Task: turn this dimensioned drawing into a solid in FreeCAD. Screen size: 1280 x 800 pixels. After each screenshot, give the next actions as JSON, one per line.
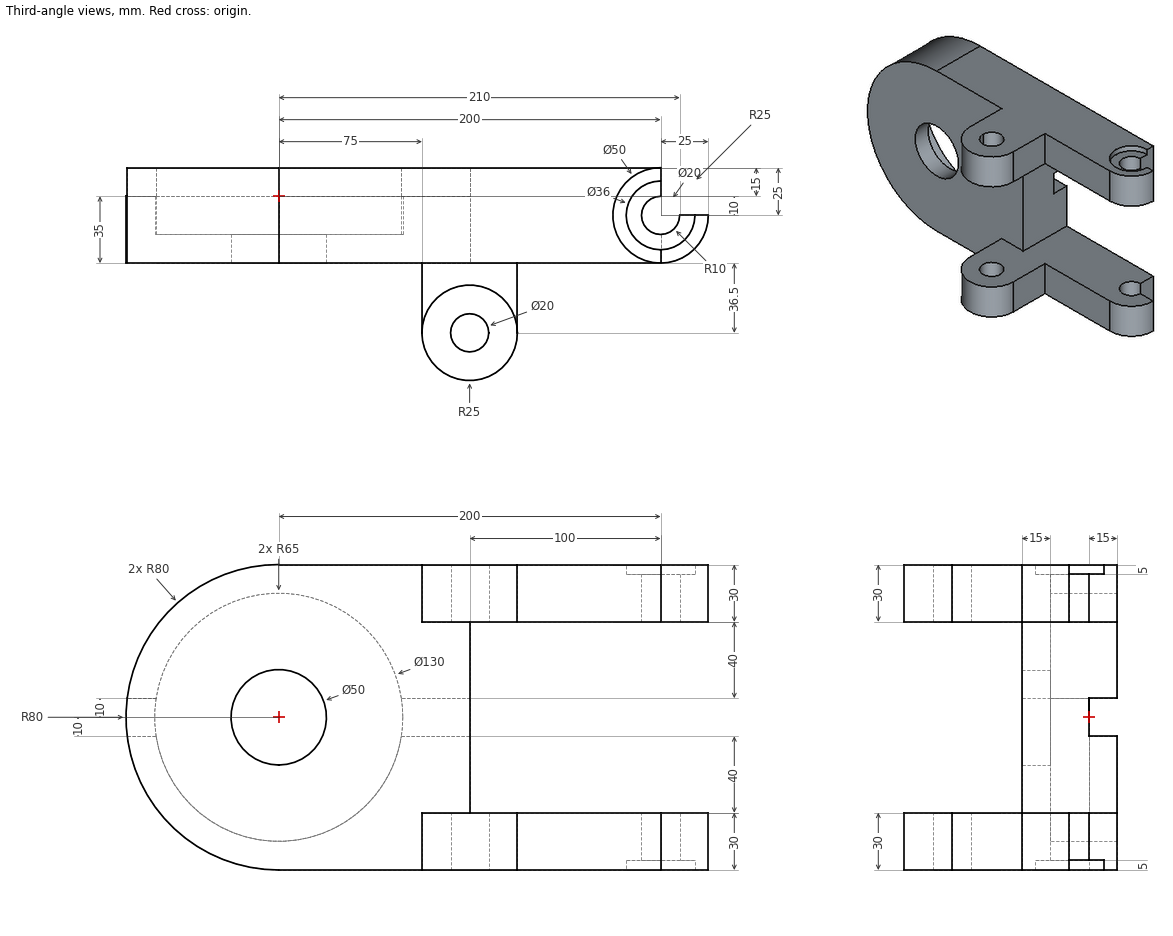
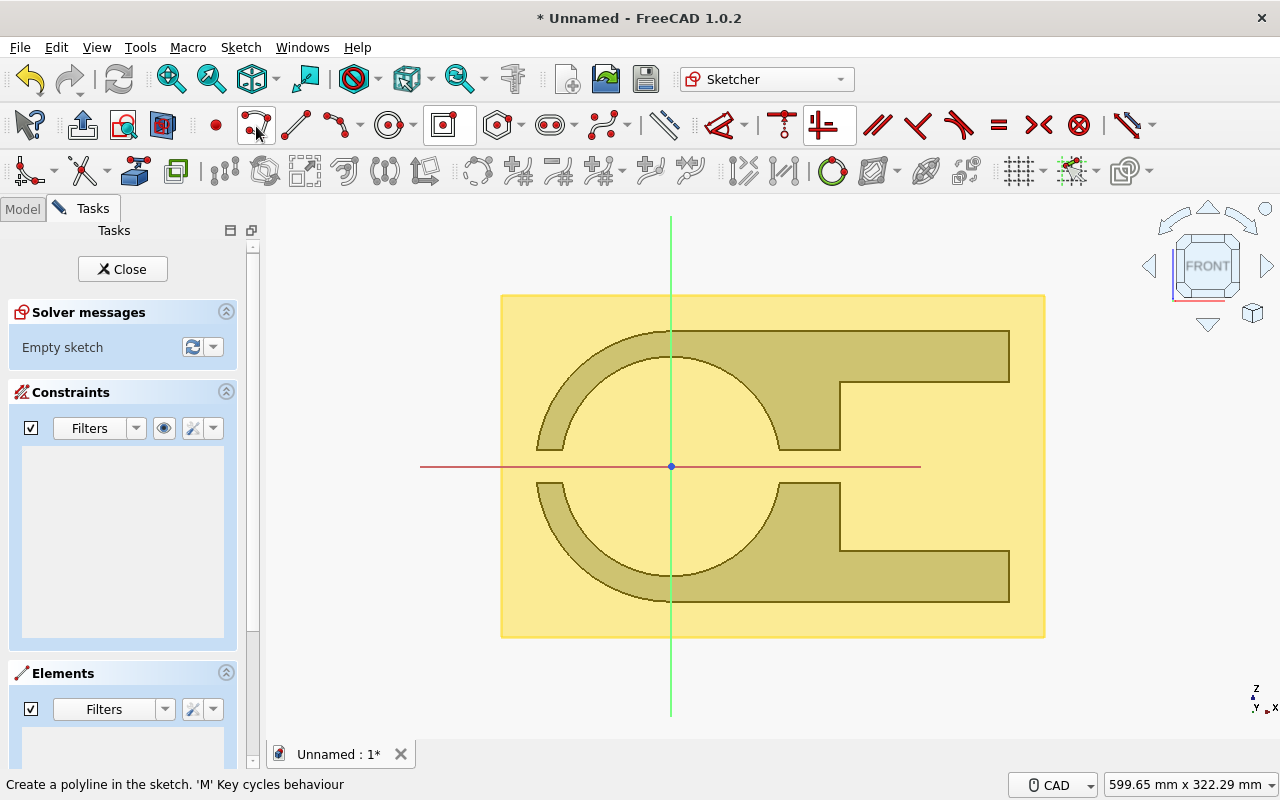
{"action": "left_click", "coordinate": [671, 602]}
{"action": "left_click", "coordinate": [1009, 602]}
{"action": "left_click", "coordinate": [1009, 551]}
{"action": "left_click", "coordinate": [840, 551]}
{"action": "left_click", "coordinate": [840, 382]}
{"action": "left_click", "coordinate": [1009, 382]}
{"action": "left_click", "coordinate": [1009, 331]}
{"action": "left_click", "coordinate": [671, 331]}
{"action": "right_click", "coordinate": [671, 331]}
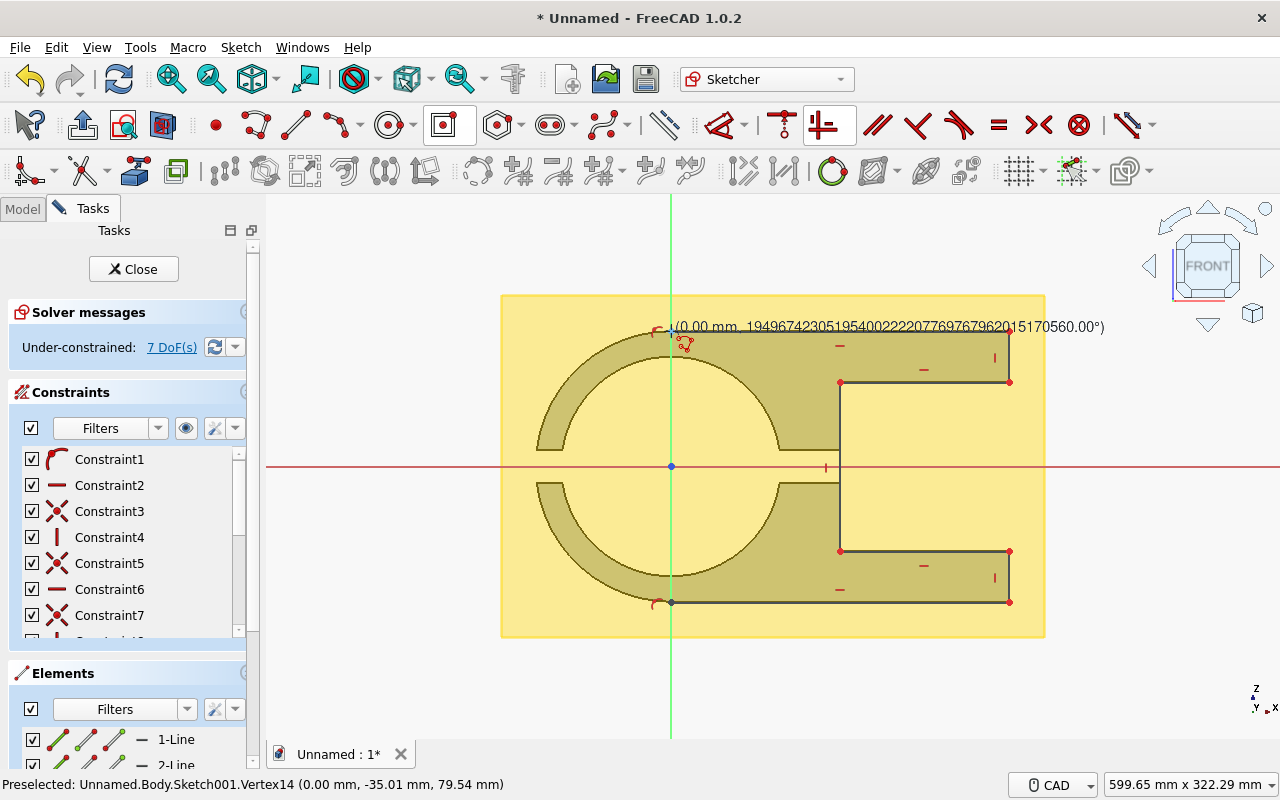
{"action": "left_click", "coordinate": [336, 126]}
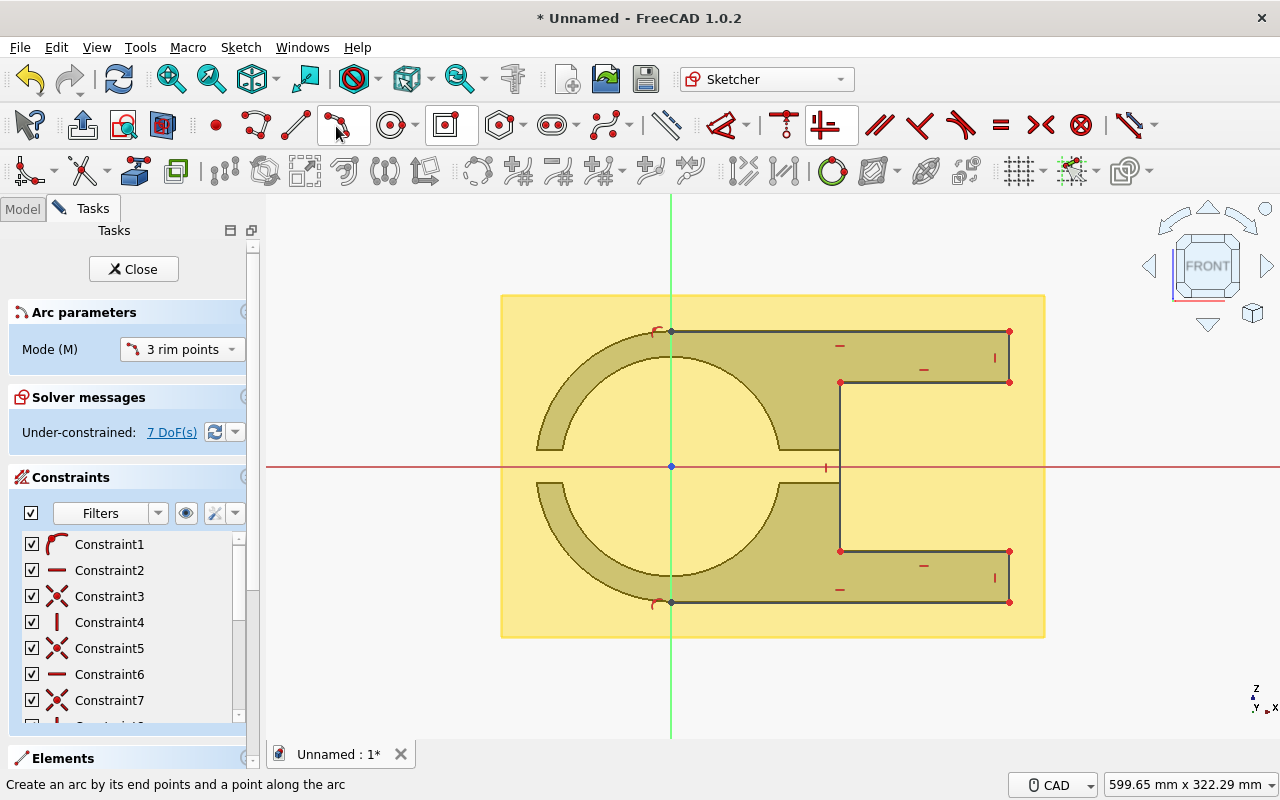
{"action": "left_click", "coordinate": [671, 332]}
{"action": "left_click", "coordinate": [671, 603]}
{"action": "left_click", "coordinate": [542, 425]}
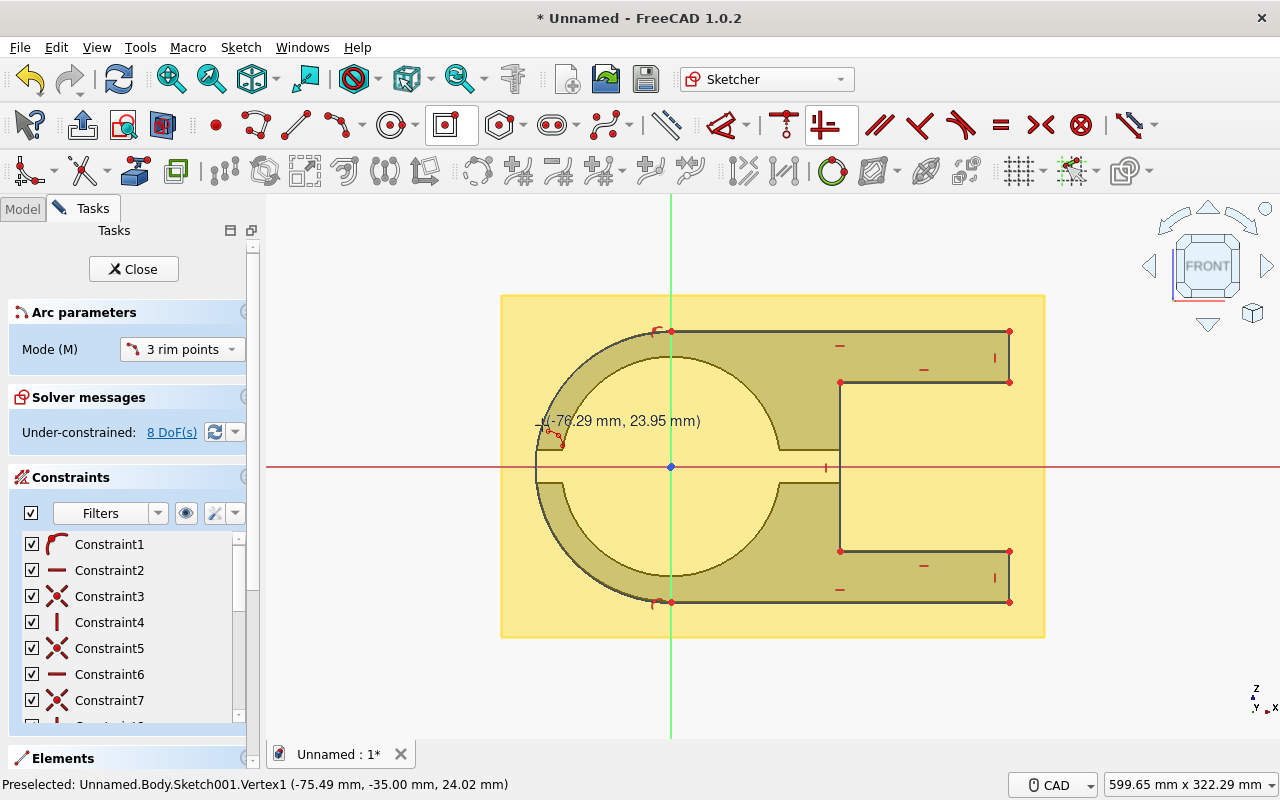
{"action": "left_click", "coordinate": [392, 126]}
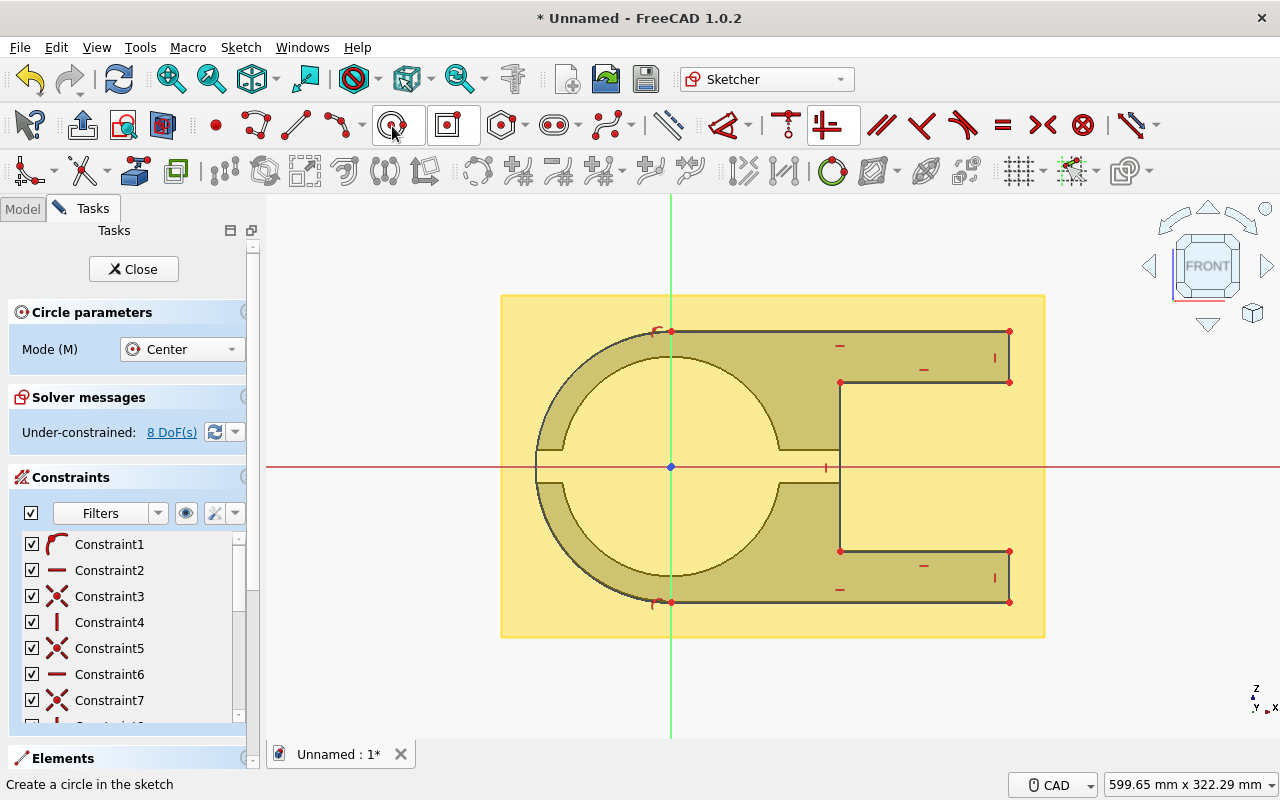
{"action": "left_click", "coordinate": [671, 466]}
{"action": "left_click", "coordinate": [749, 389]}
{"action": "key", "text": "Escape"}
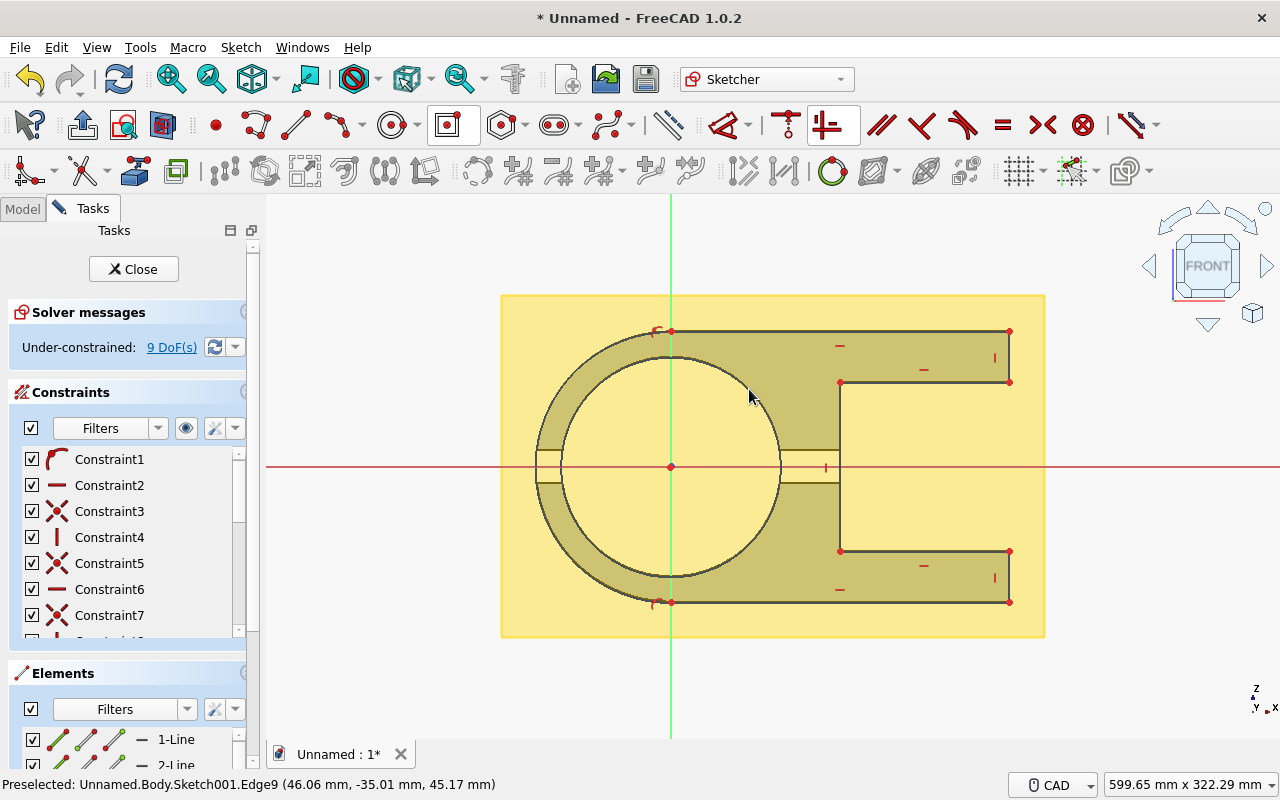
{"action": "left_click_drag", "start_coordinate": [661, 456], "coordinate": [681, 478]}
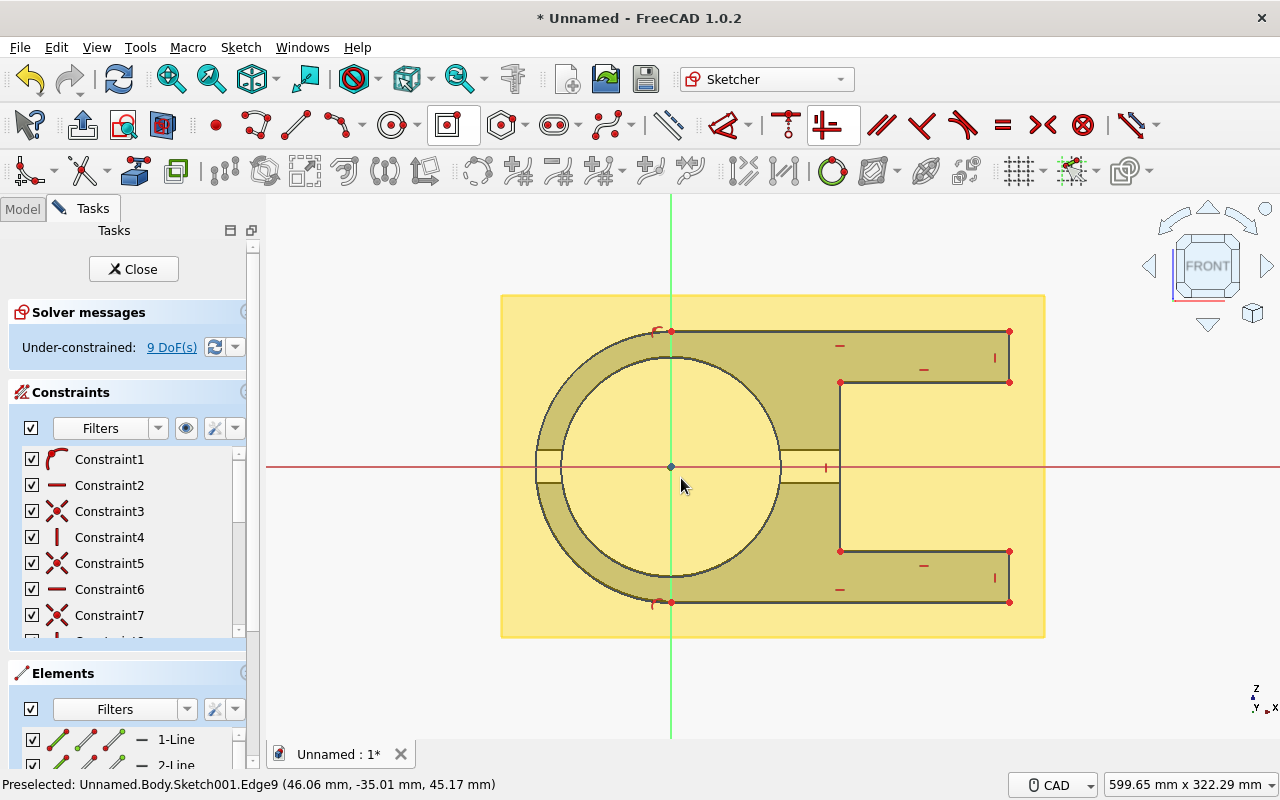
{"action": "left_click", "coordinate": [786, 126]}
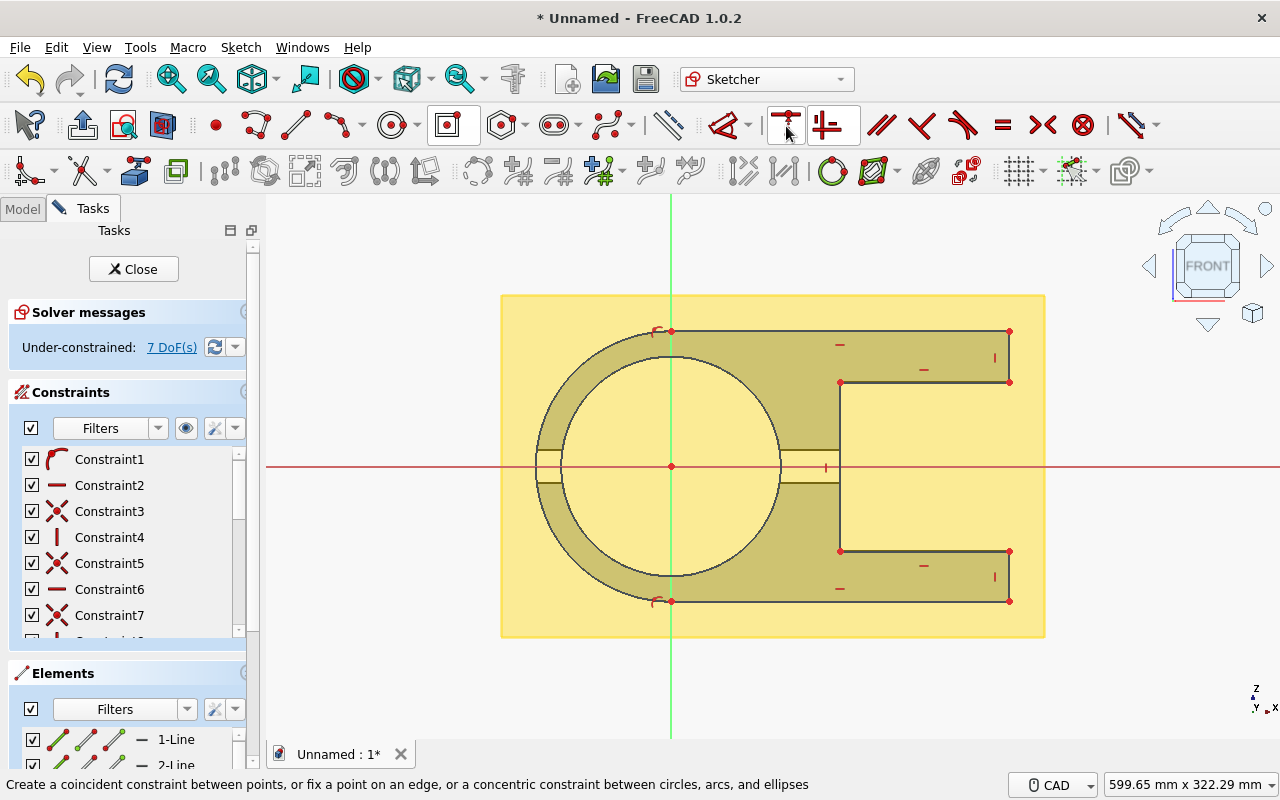
{"action": "left_click", "coordinate": [724, 126]}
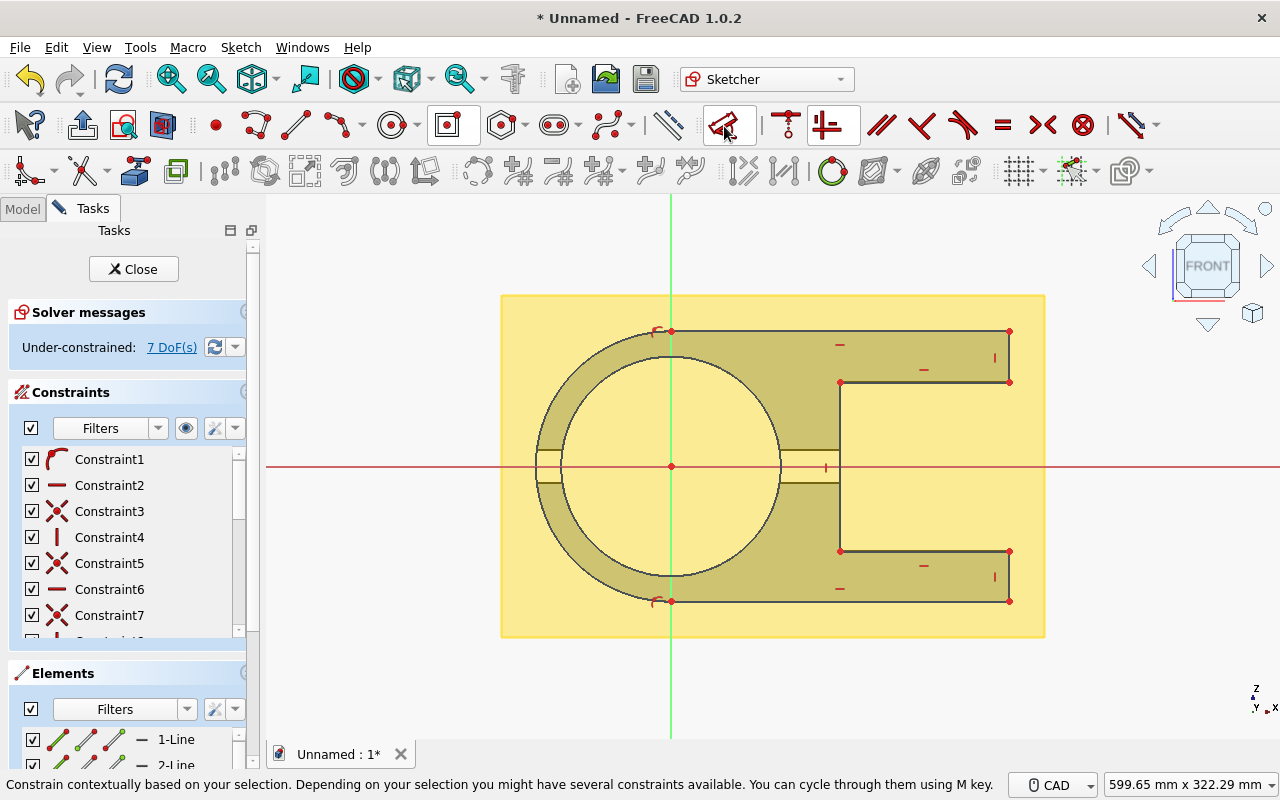
{"action": "left_click", "coordinate": [562, 387]}
{"action": "left_click", "coordinate": [536, 368]}